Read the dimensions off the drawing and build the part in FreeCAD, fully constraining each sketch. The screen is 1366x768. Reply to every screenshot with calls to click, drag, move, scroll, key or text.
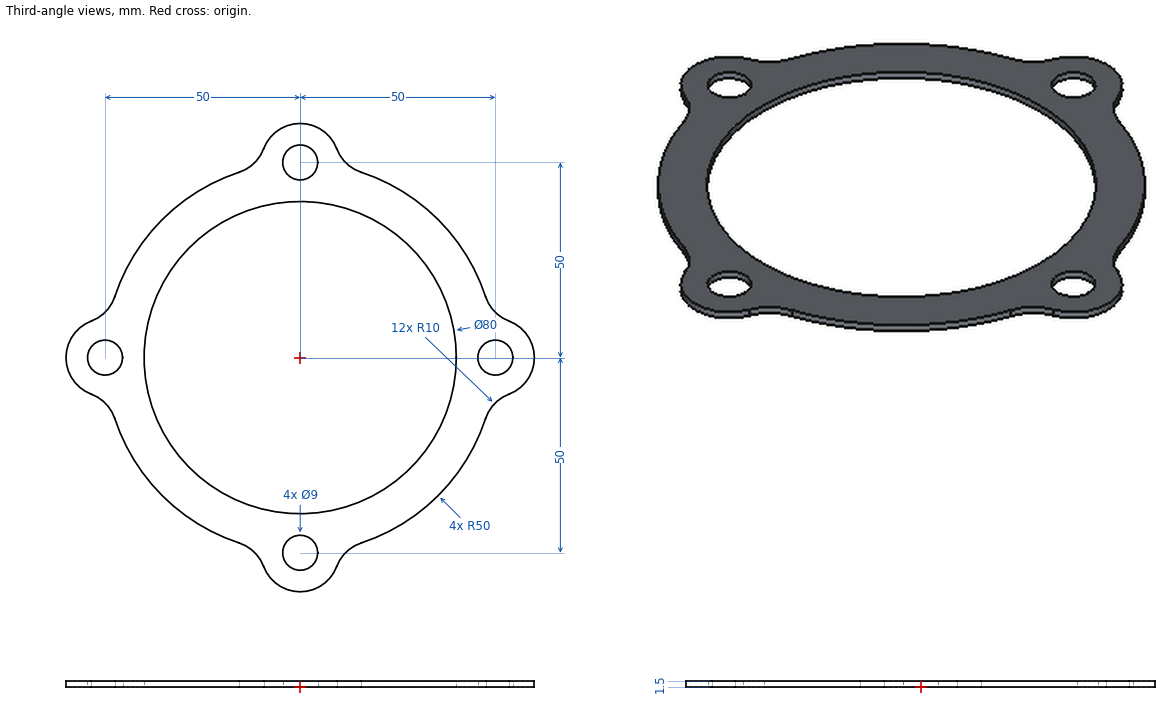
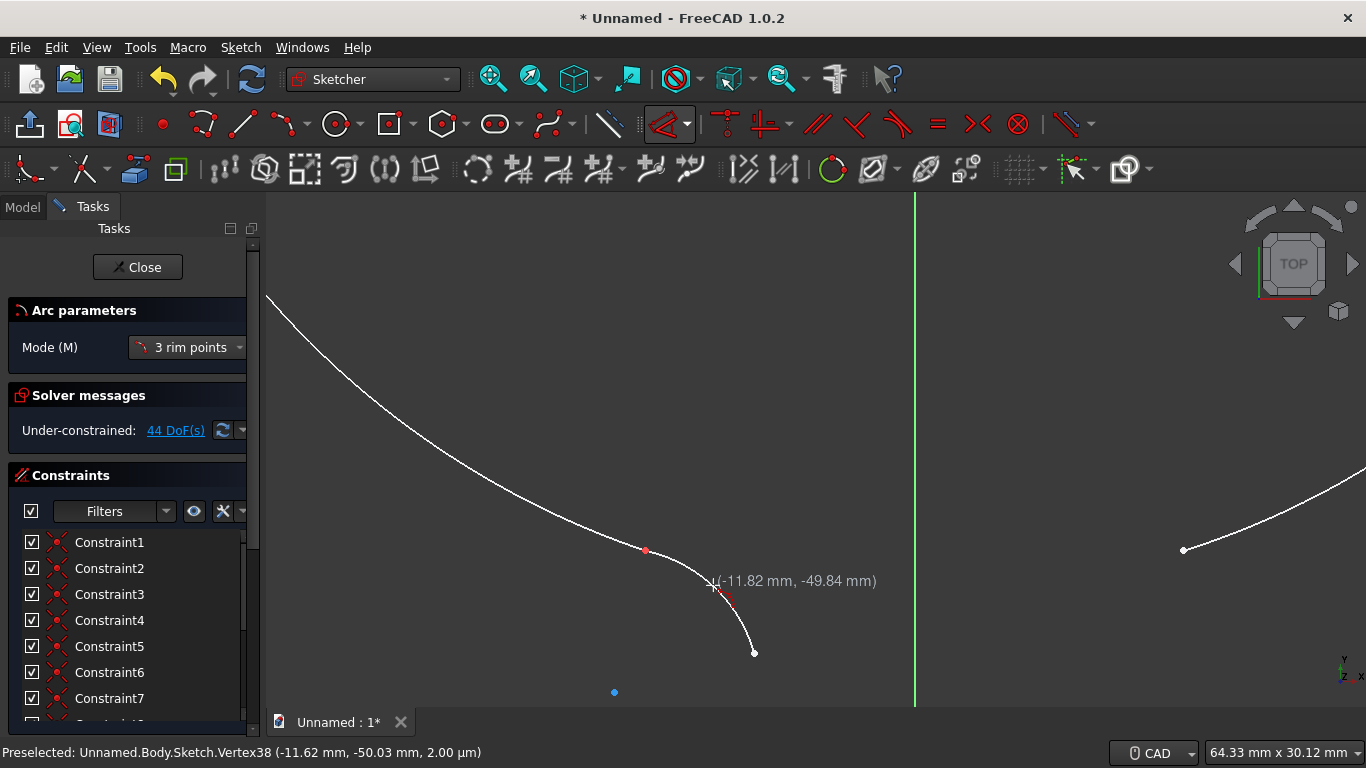
scroll(714, 591, down, 9)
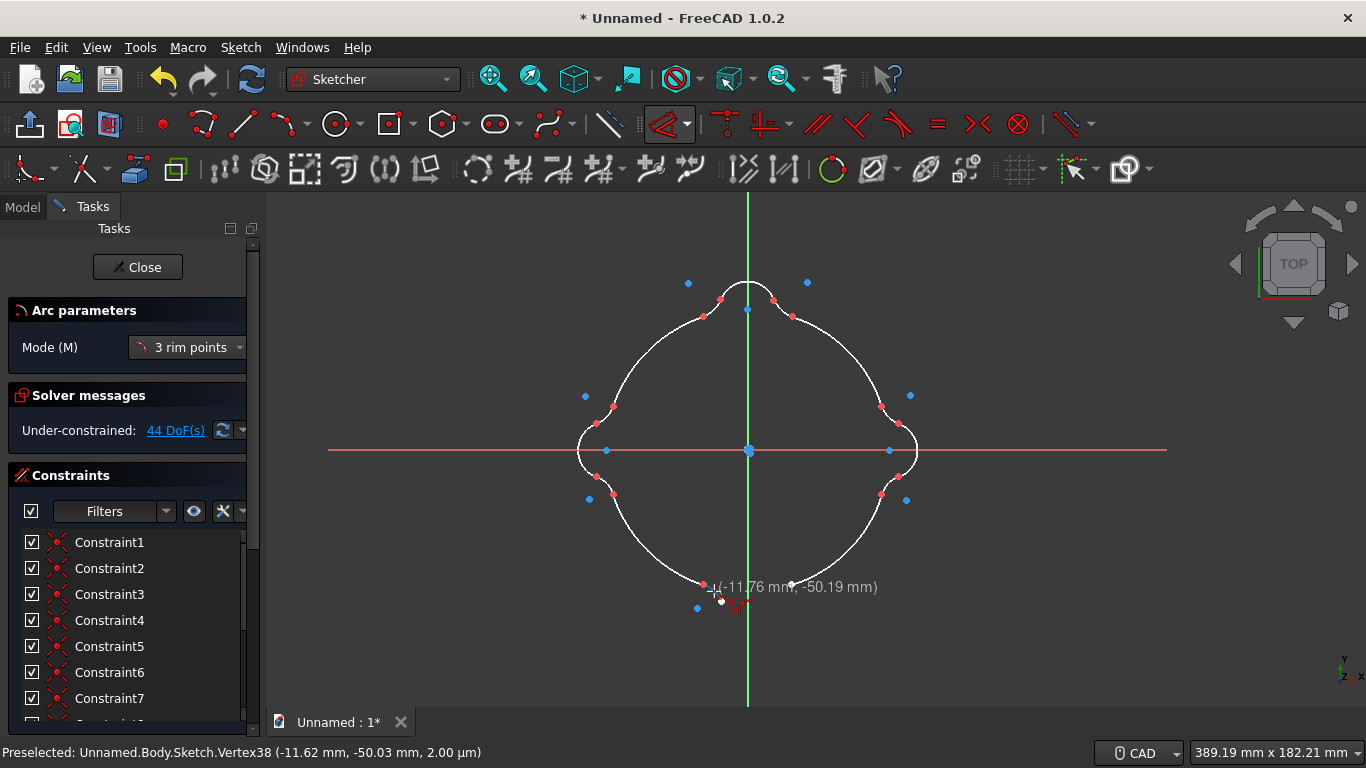
click(721, 602)
click(774, 601)
click(761, 616)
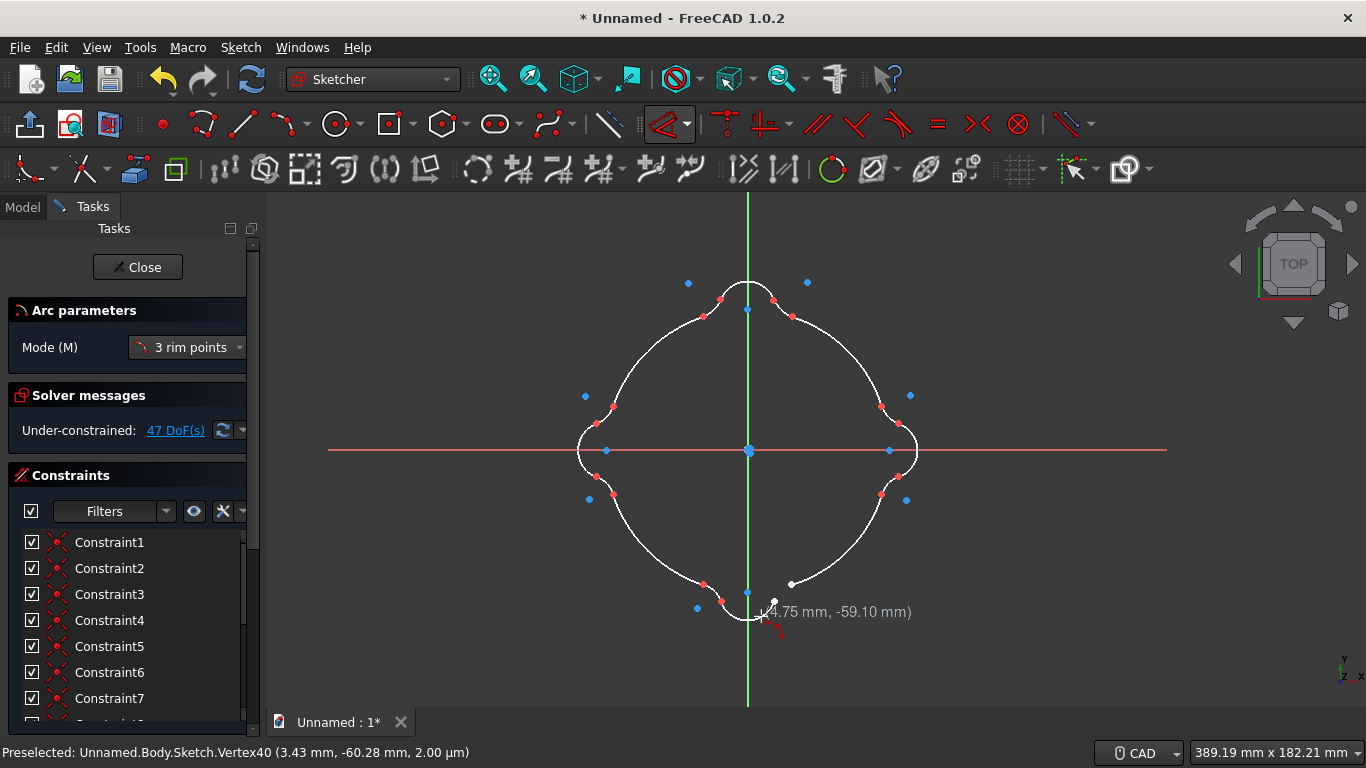
click(774, 602)
click(792, 585)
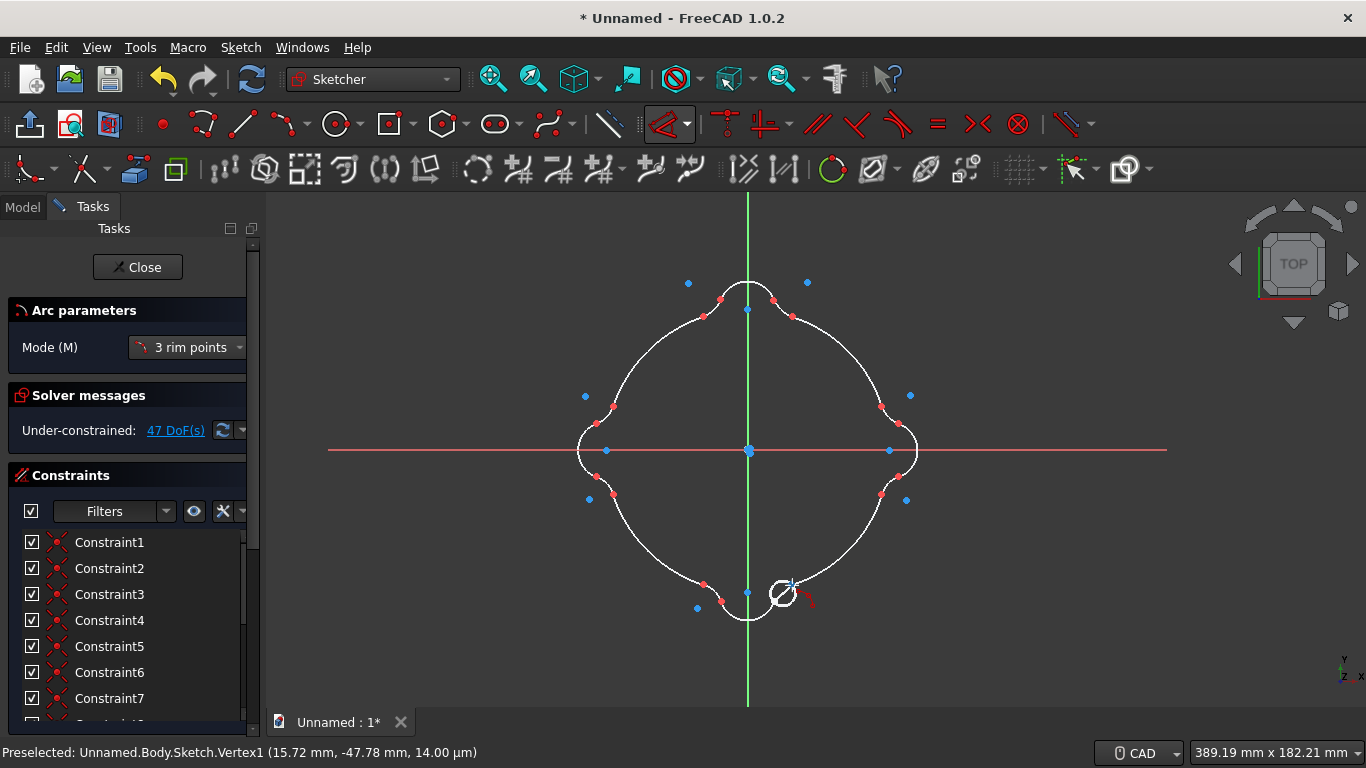
scroll(781, 591, up, 9)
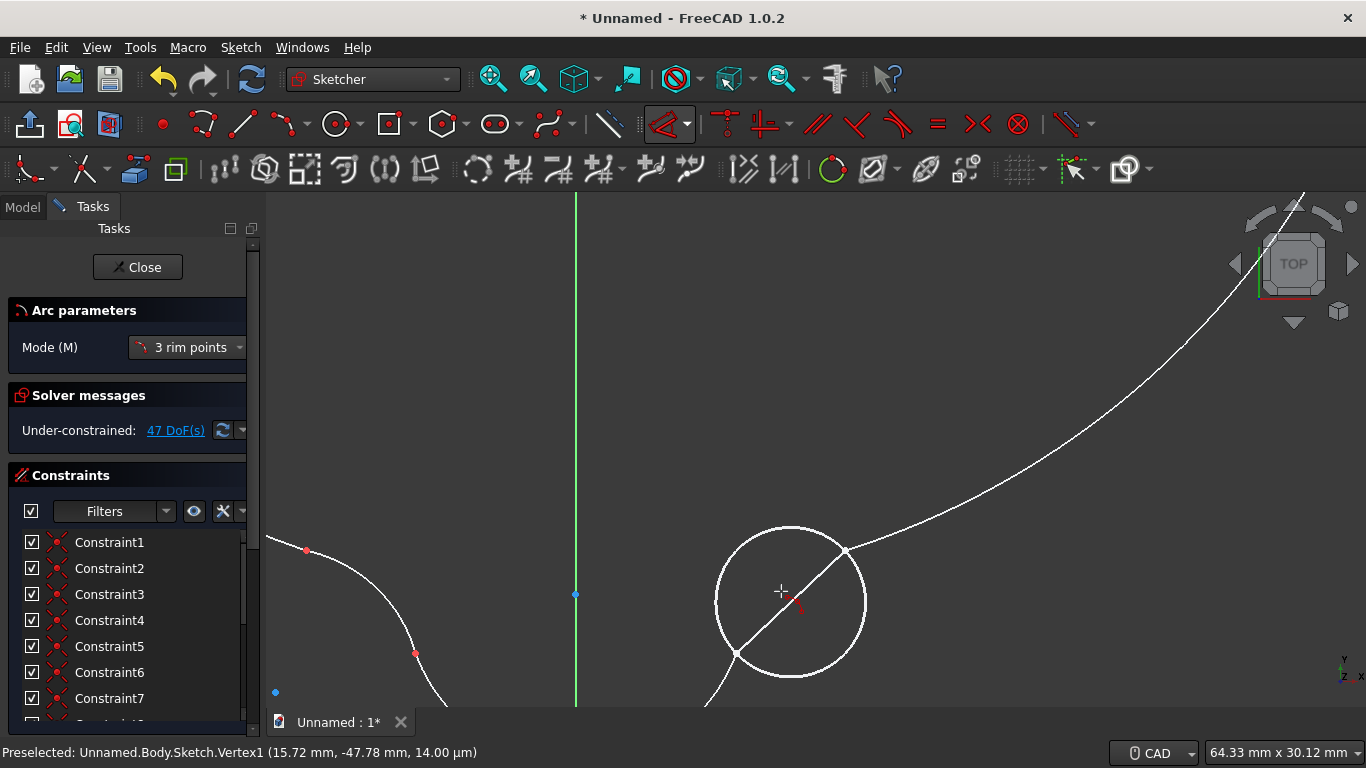
click(778, 585)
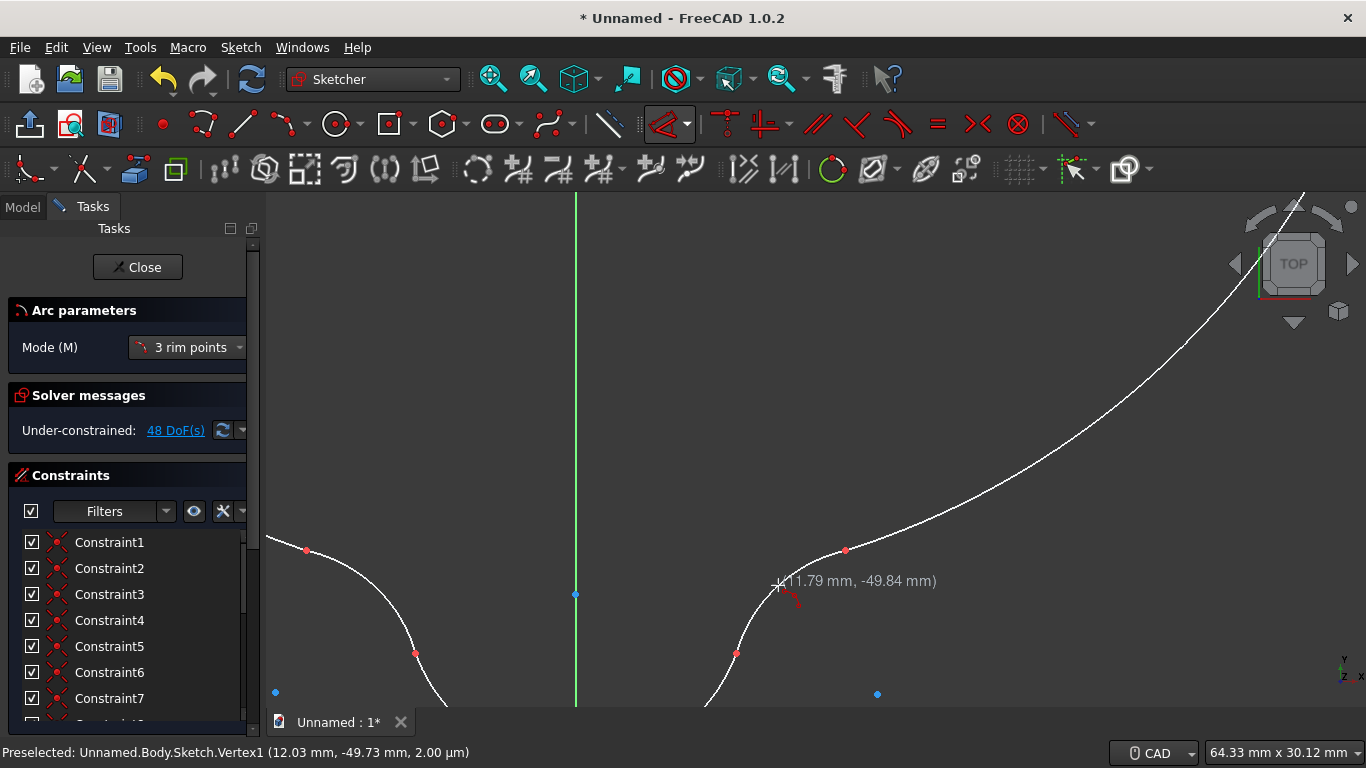
click(336, 124)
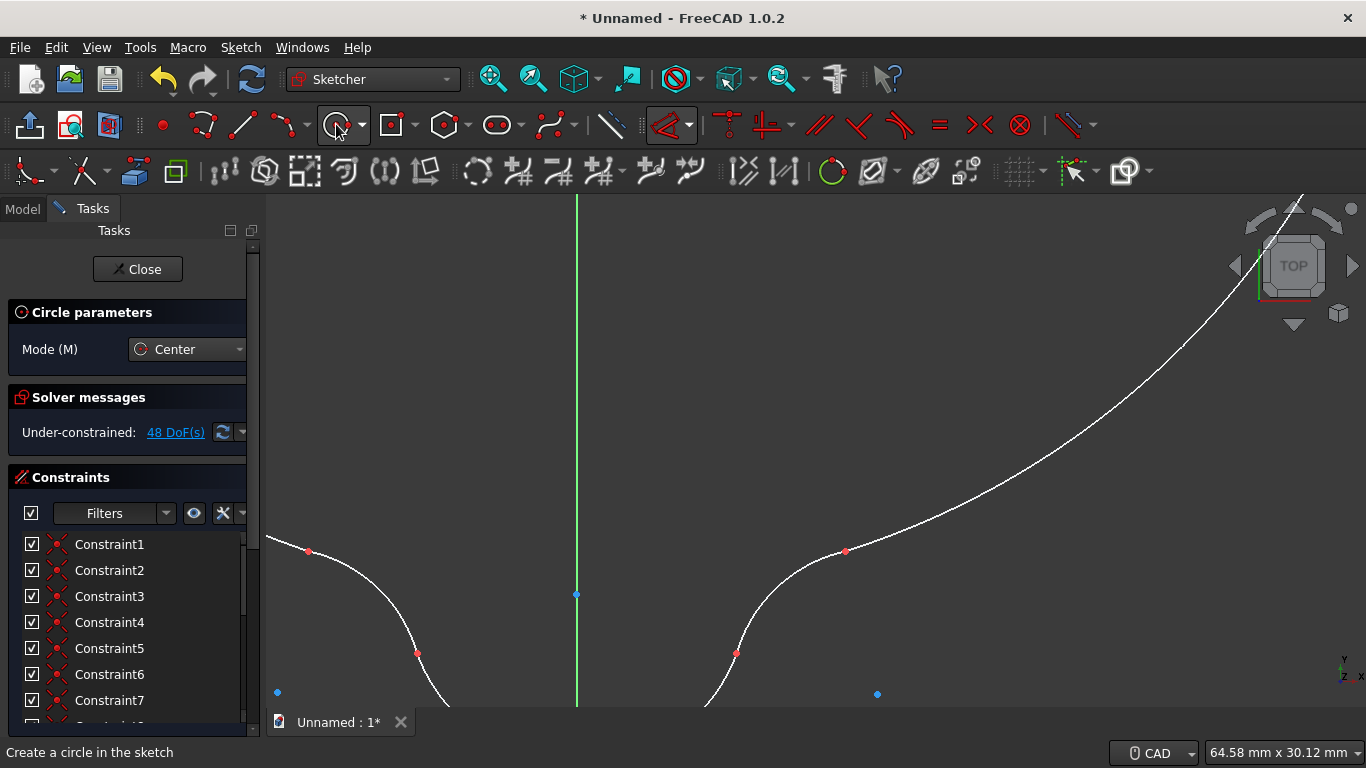
scroll(781, 592, down, 9)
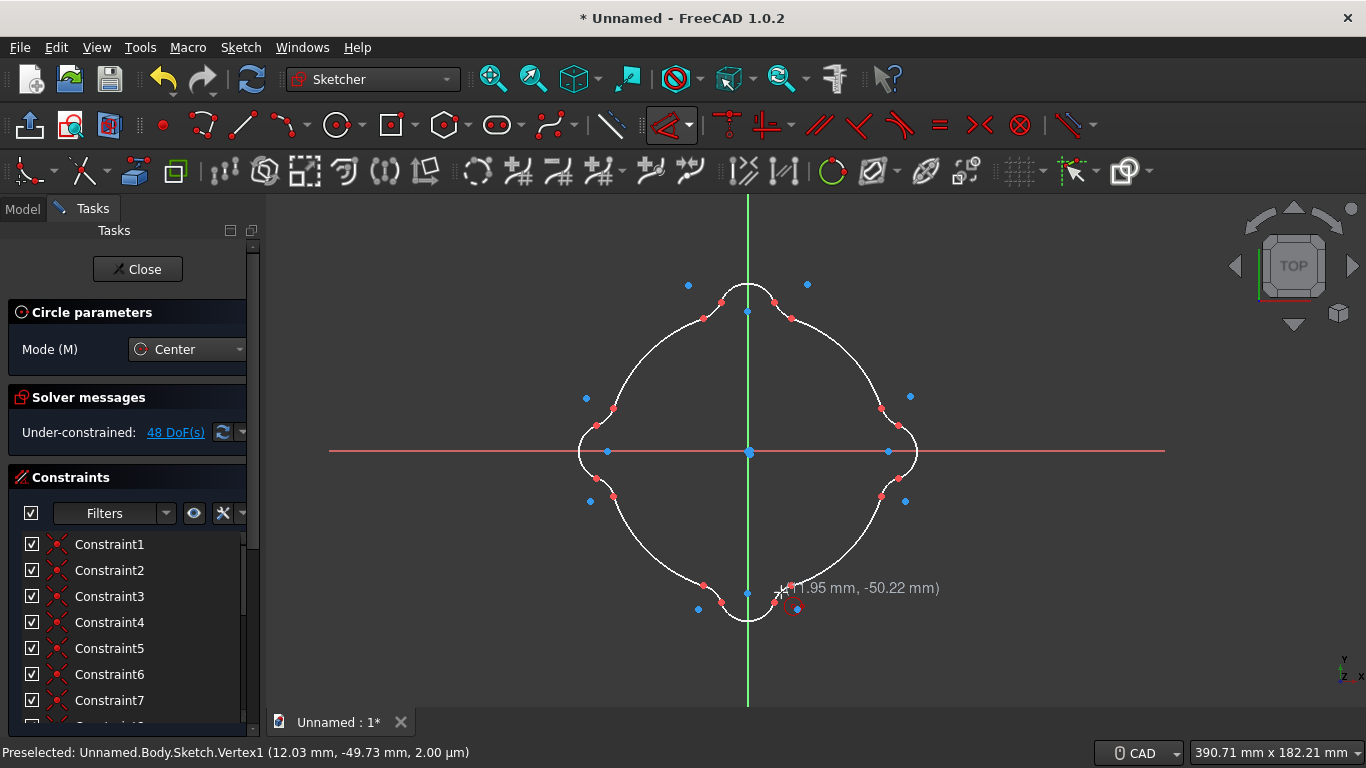
scroll(748, 592, up, 3)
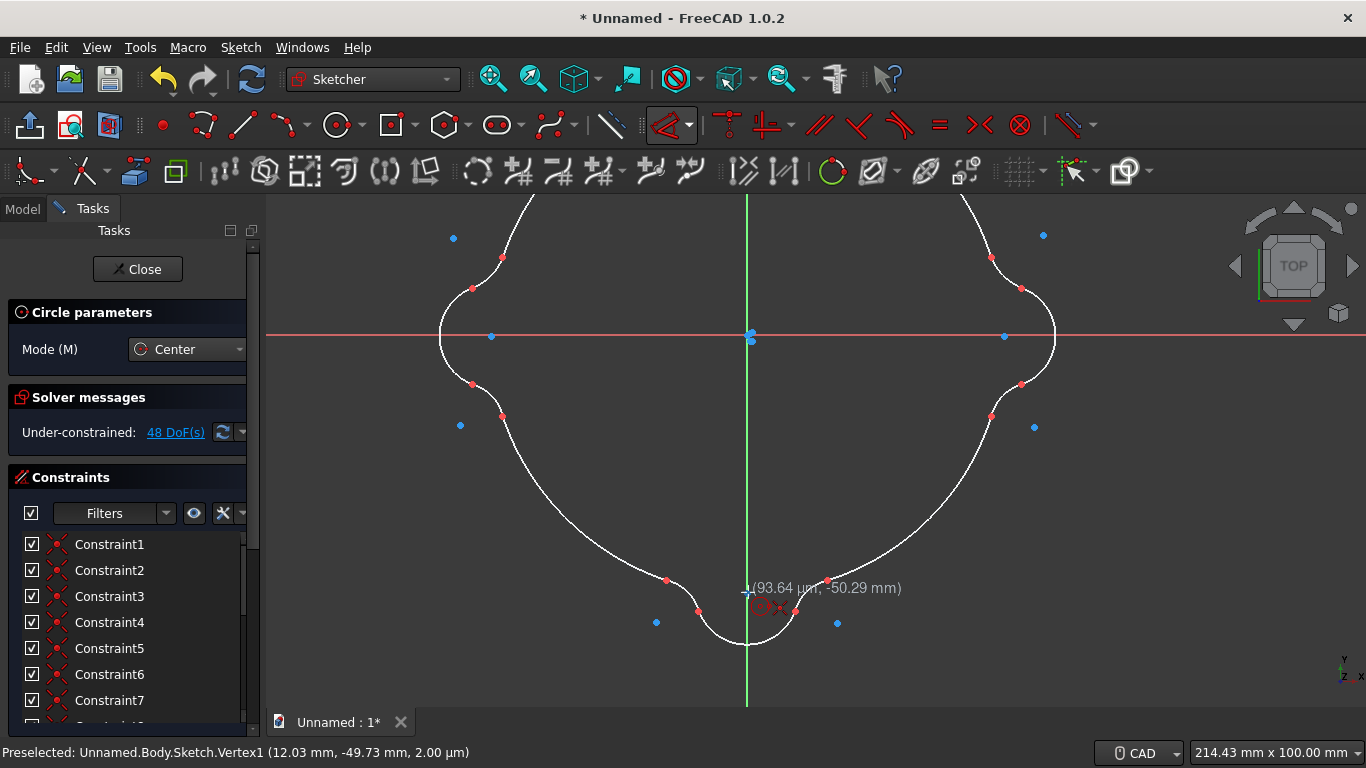
click(747, 592)
click(763, 575)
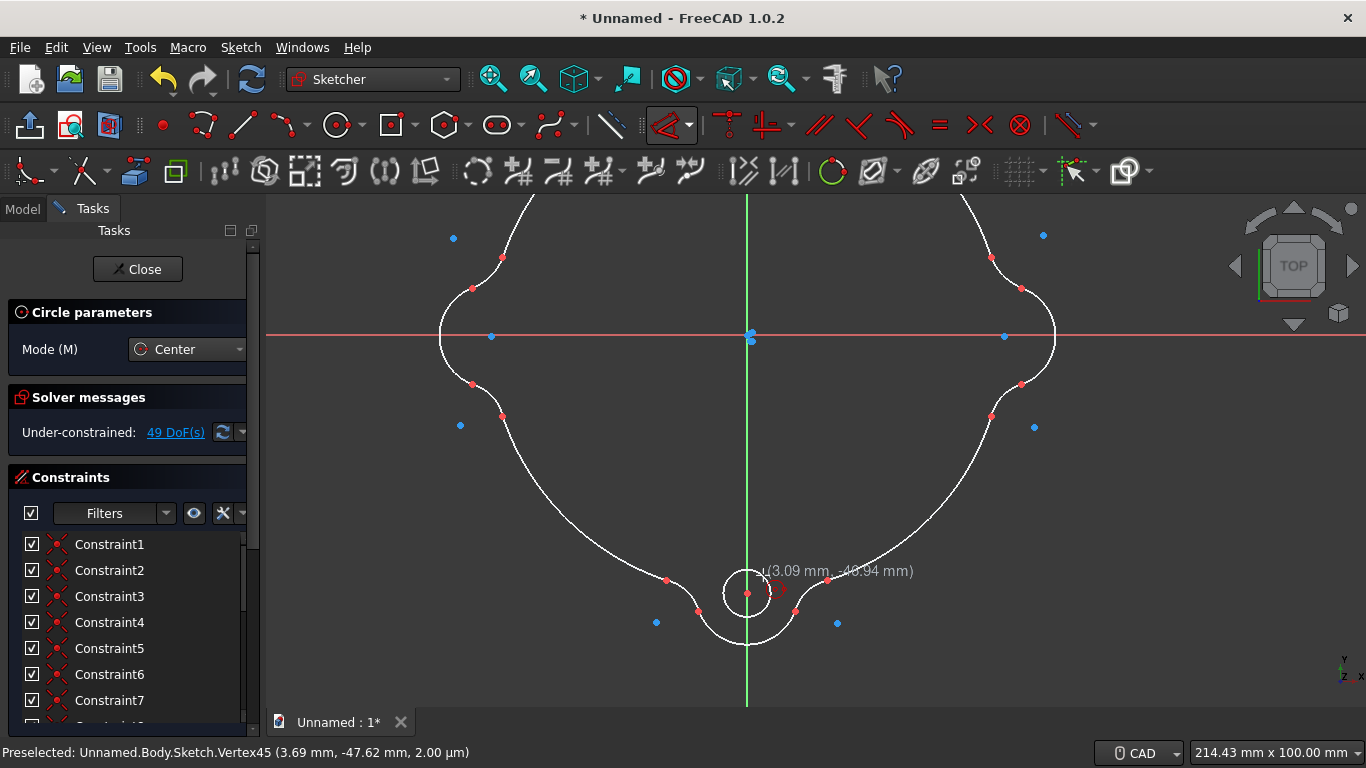
click(491, 335)
click(507, 319)